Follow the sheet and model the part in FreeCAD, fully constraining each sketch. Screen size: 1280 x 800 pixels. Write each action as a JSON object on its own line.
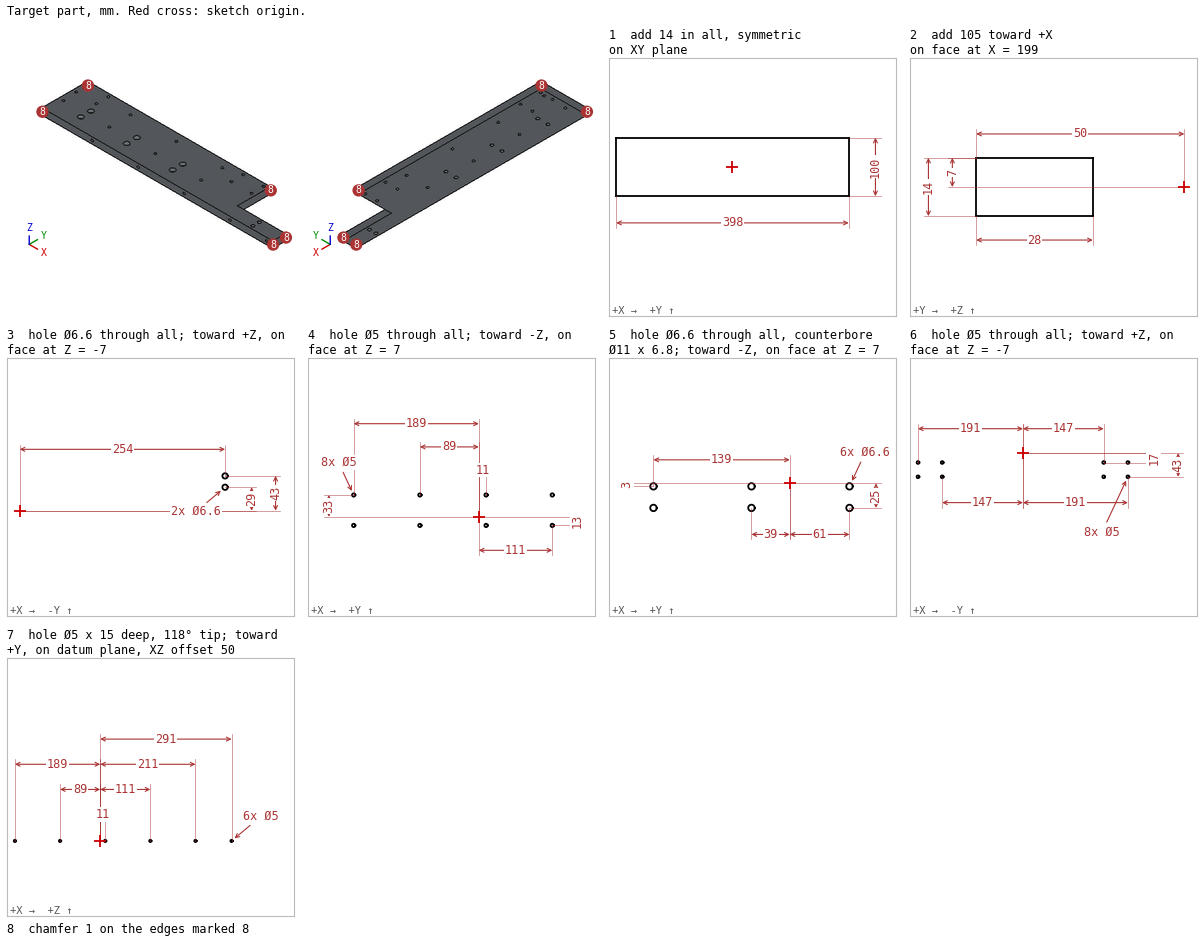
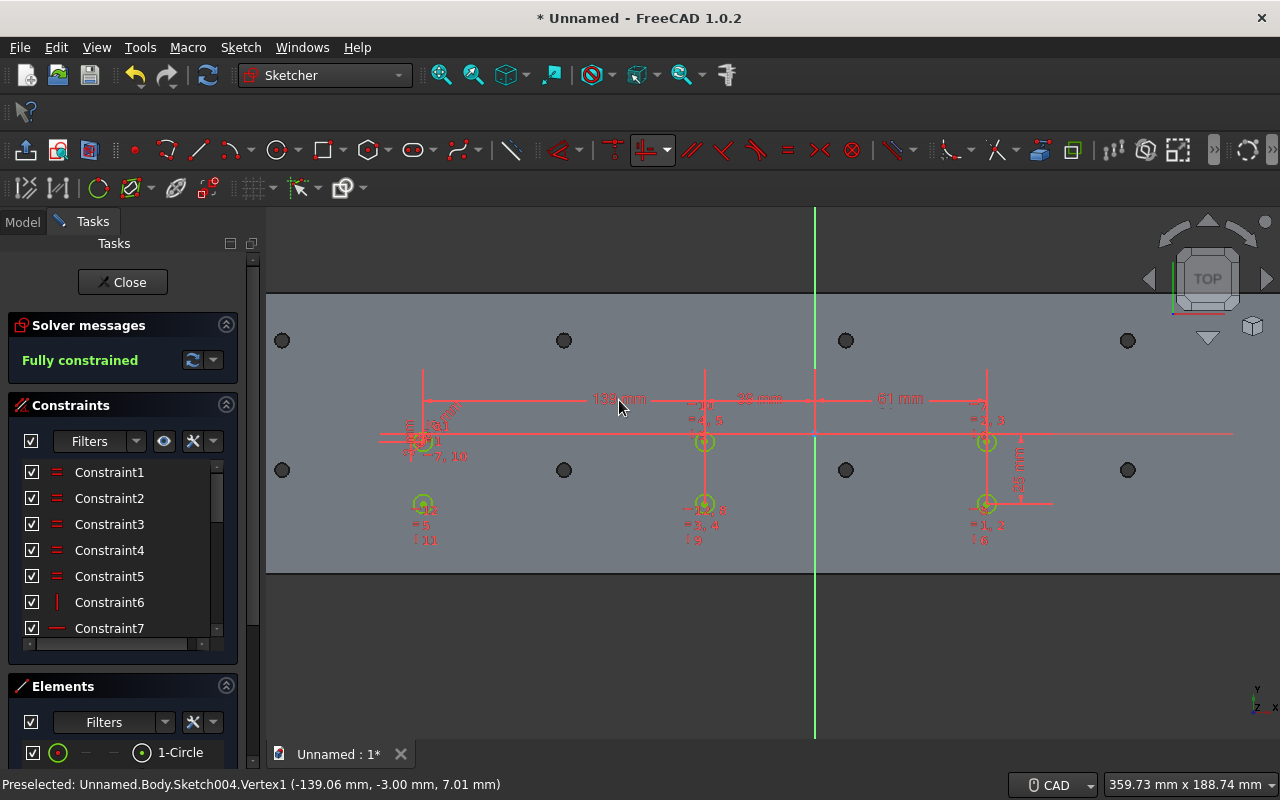
{"action": "left_click", "coordinate": [123, 282]}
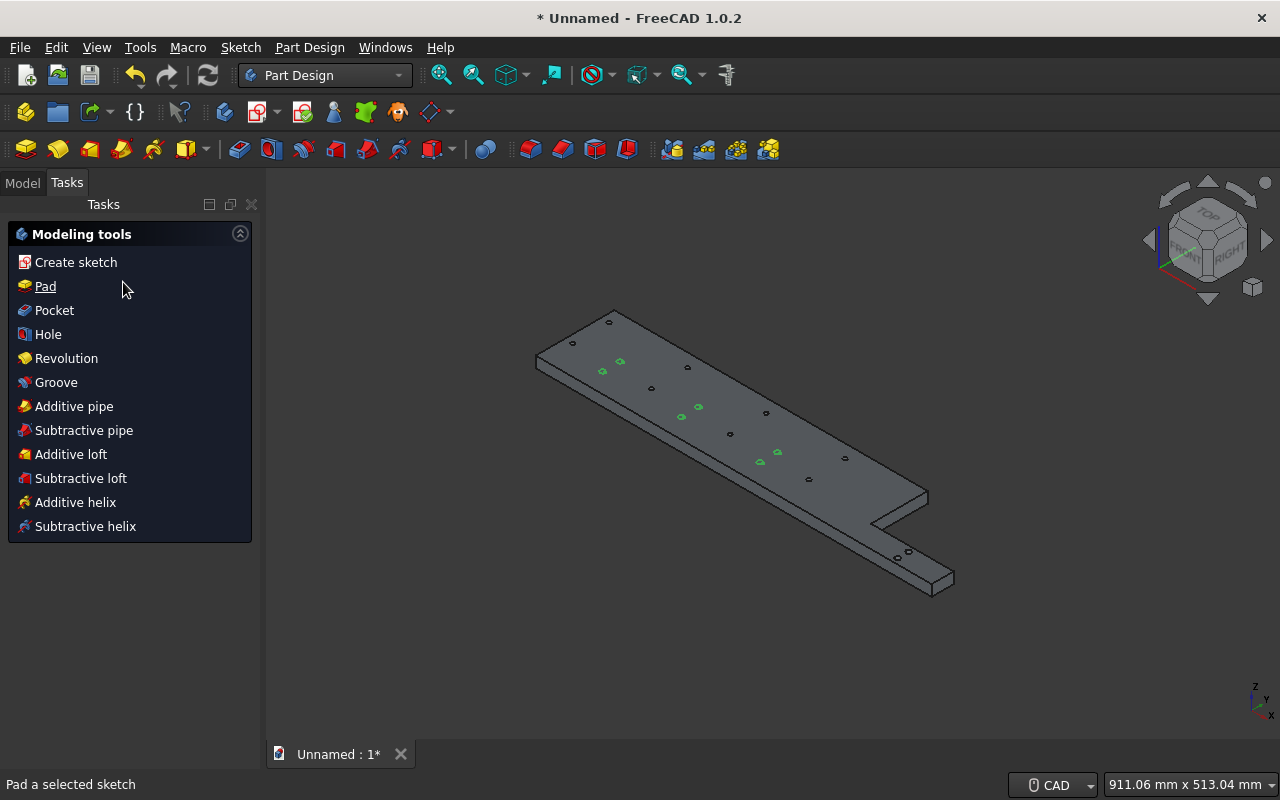
{"action": "left_click", "coordinate": [272, 150]}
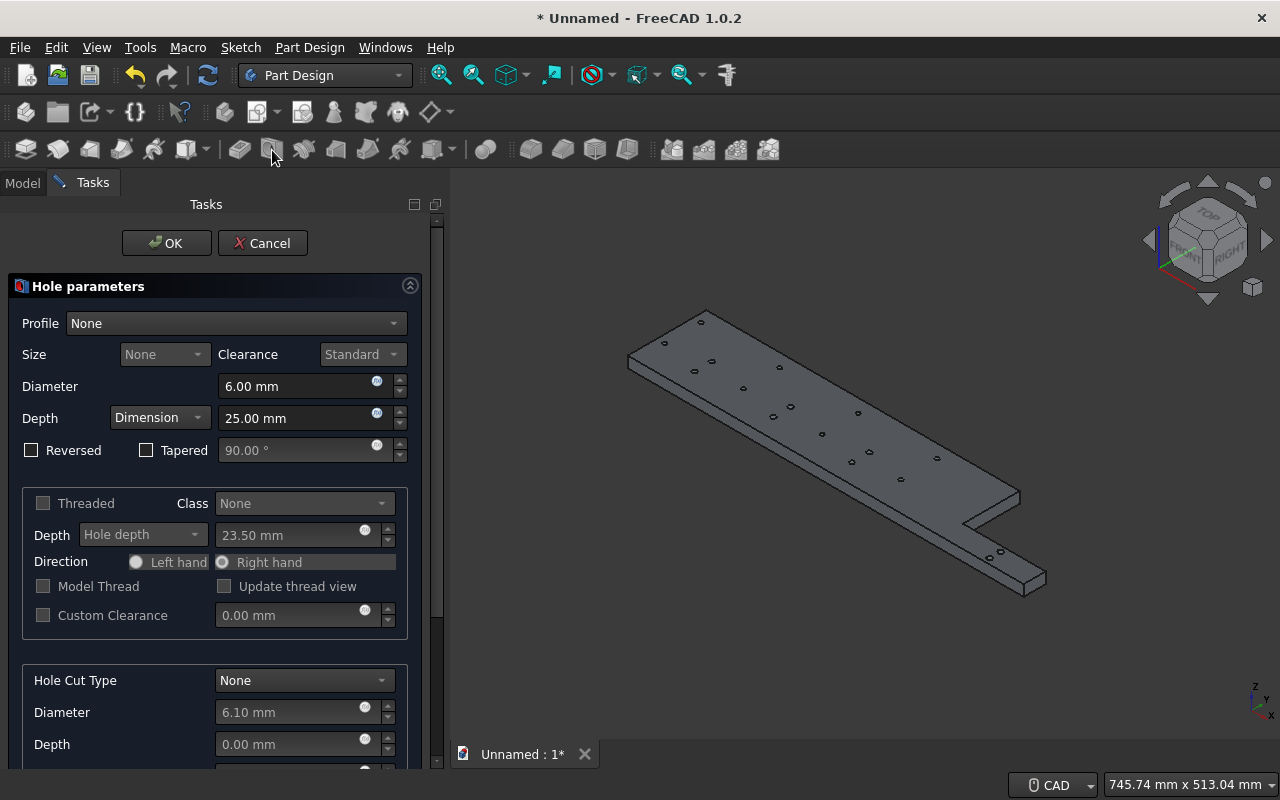
{"action": "triple_click", "coordinate": [305, 386]}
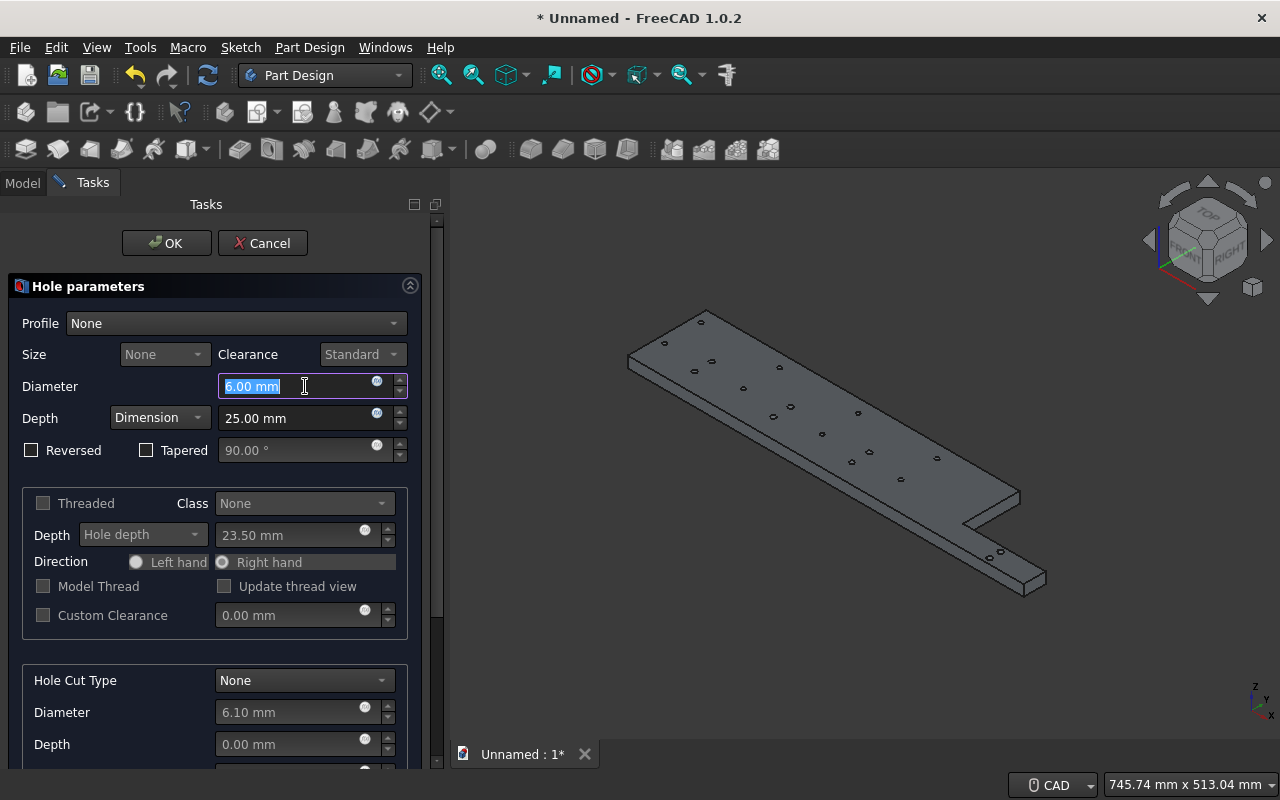
{"action": "type", "text": "6.6"}
{"action": "key", "text": "Tab"}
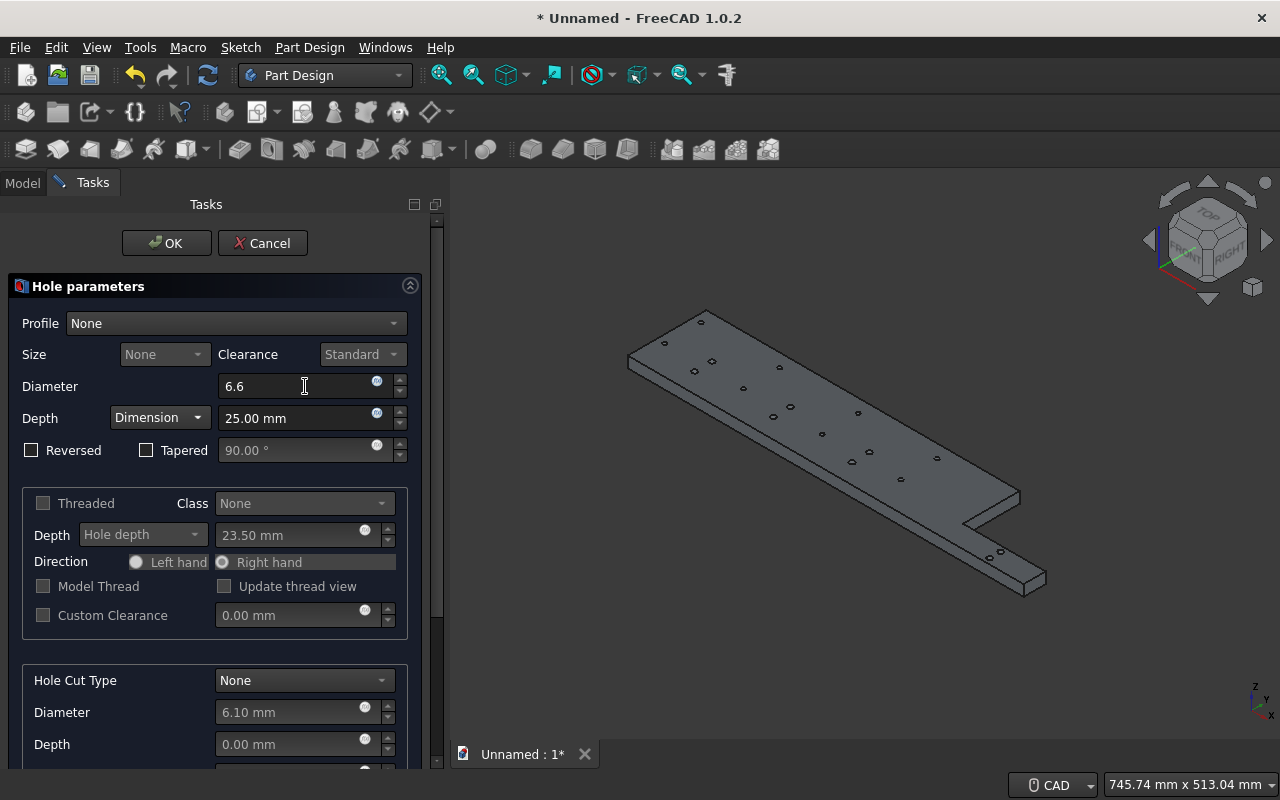
{"action": "left_click", "coordinate": [161, 418]}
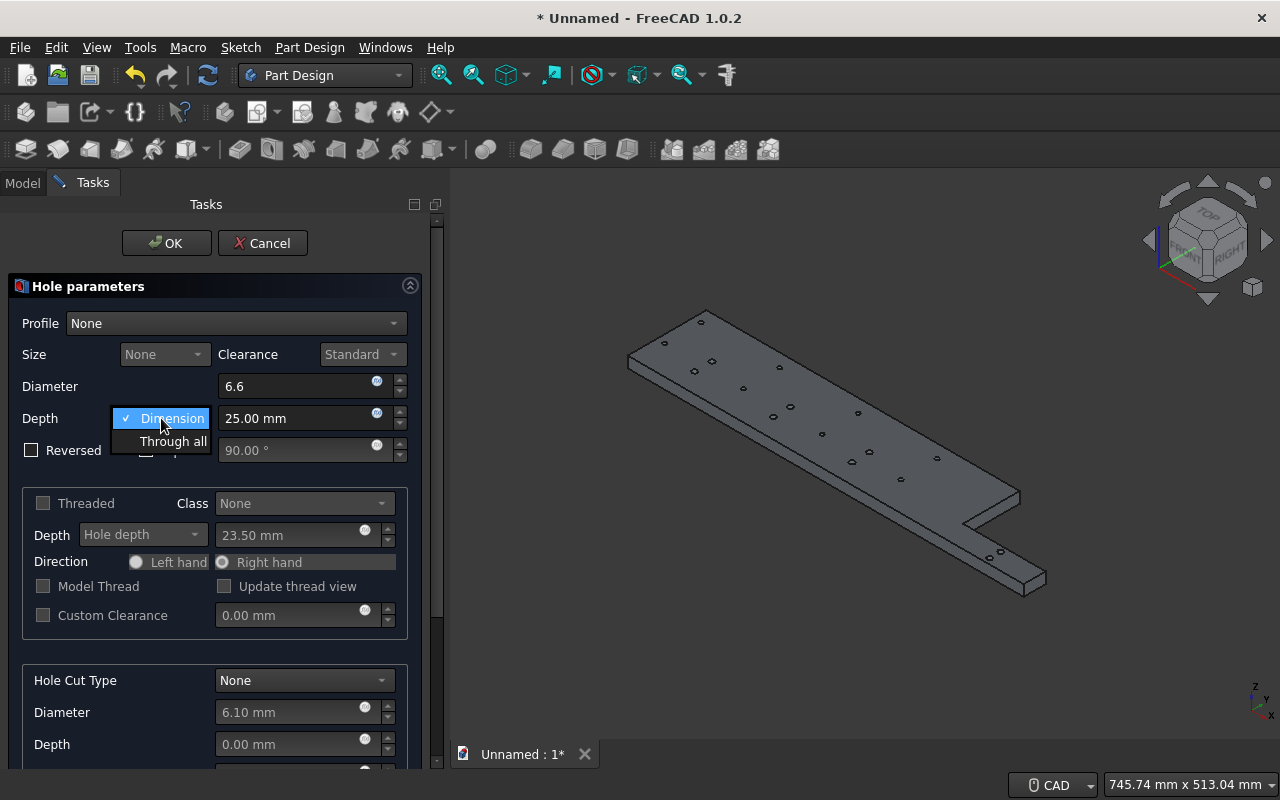
{"action": "left_click", "coordinate": [160, 442]}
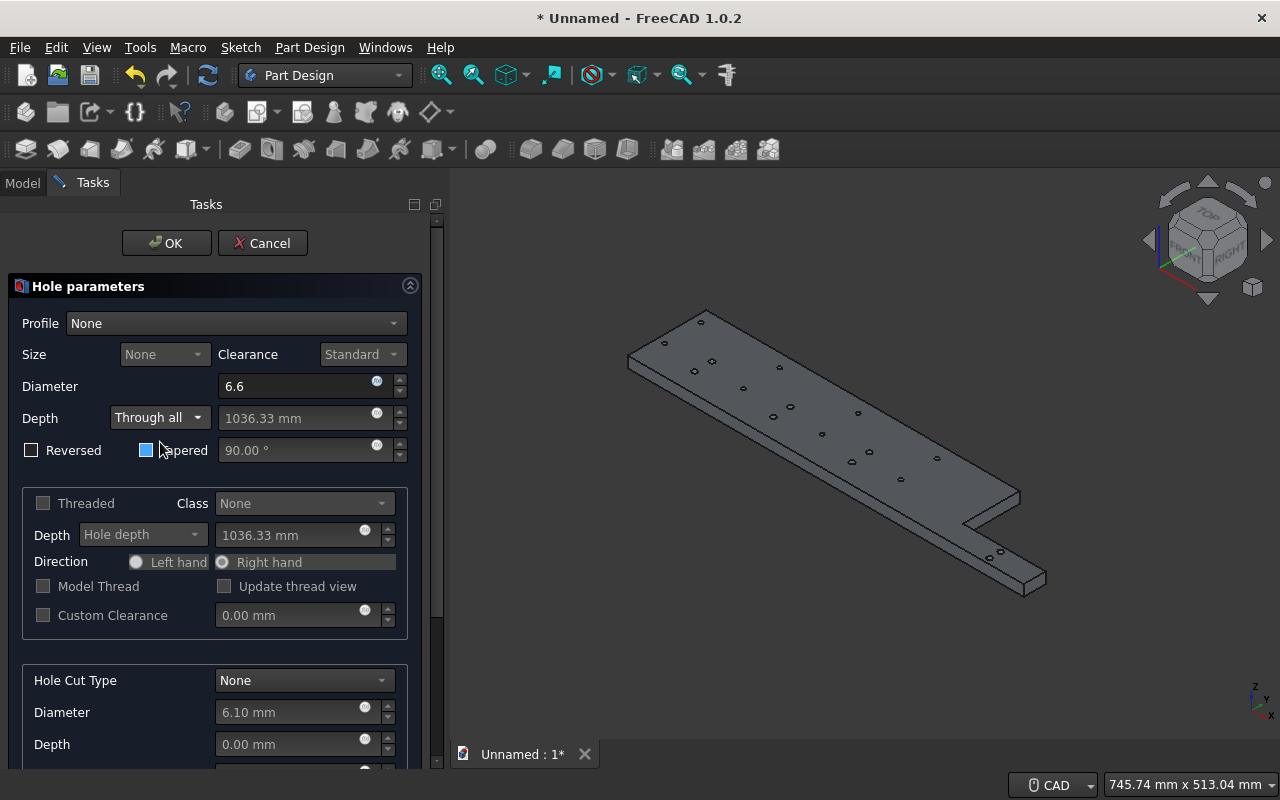
{"action": "left_click", "coordinate": [306, 680]}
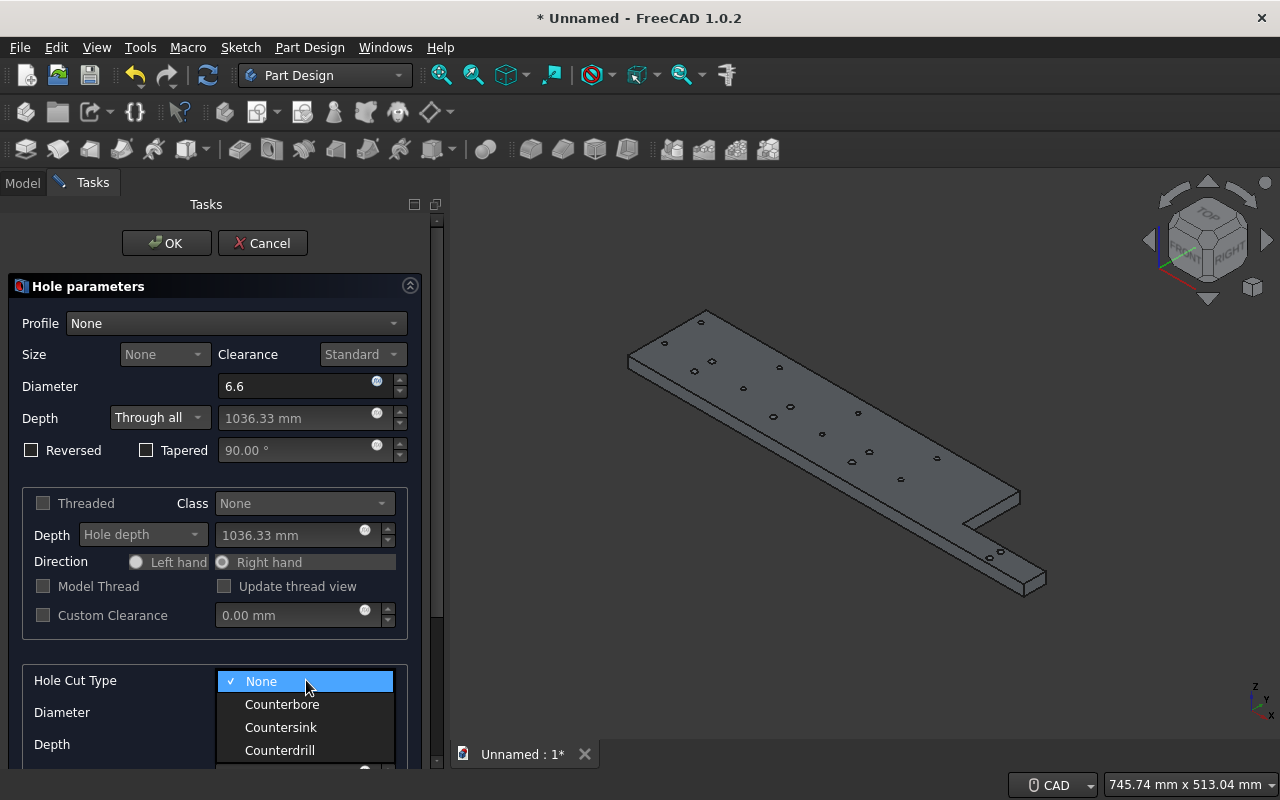
{"action": "left_click", "coordinate": [304, 704]}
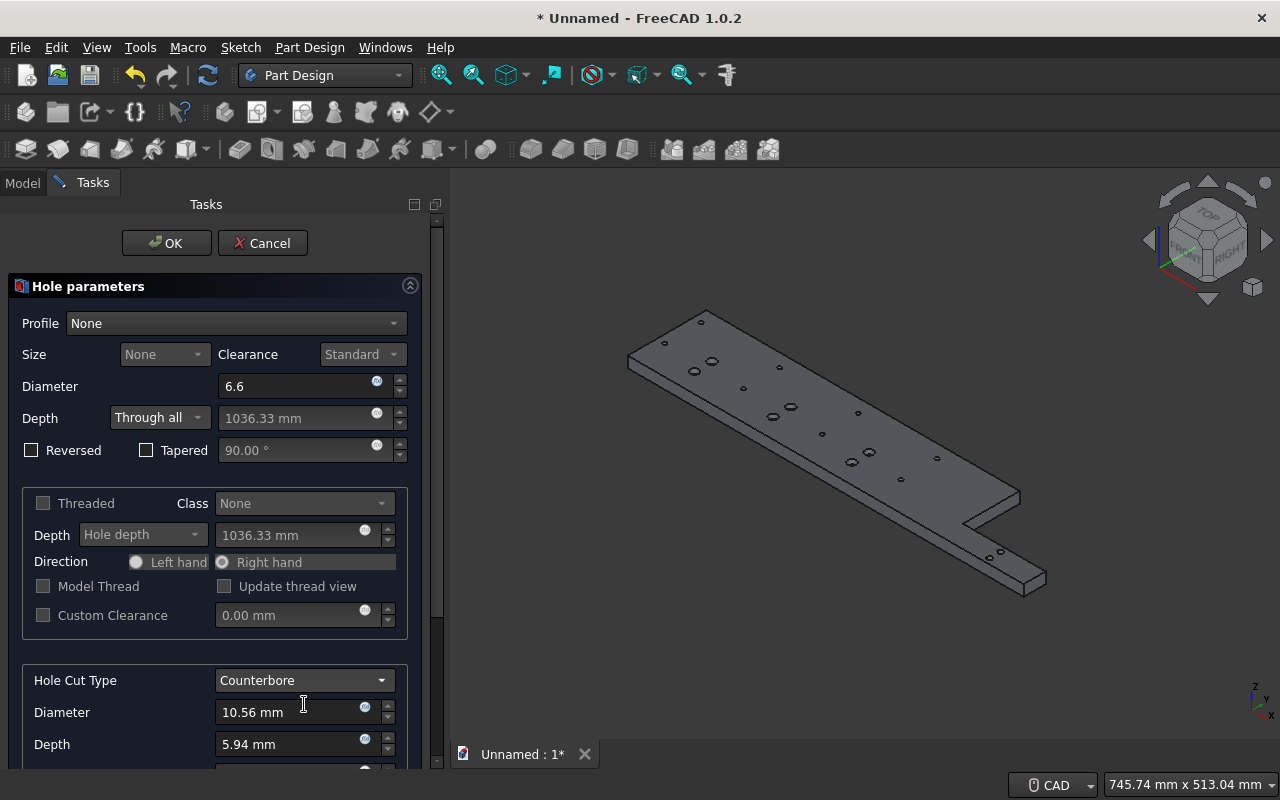
{"action": "triple_click", "coordinate": [298, 712]}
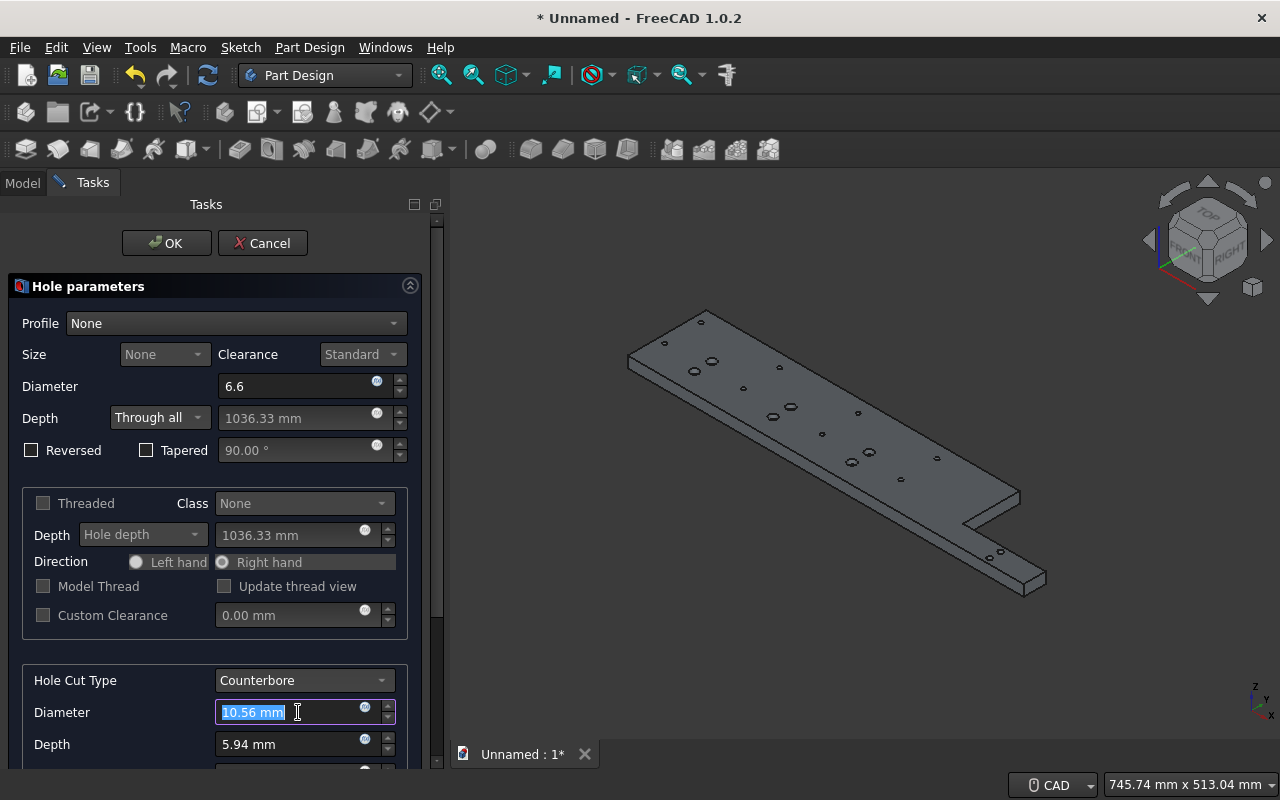
{"action": "type", "text": "11"}
{"action": "key", "text": "Tab"}